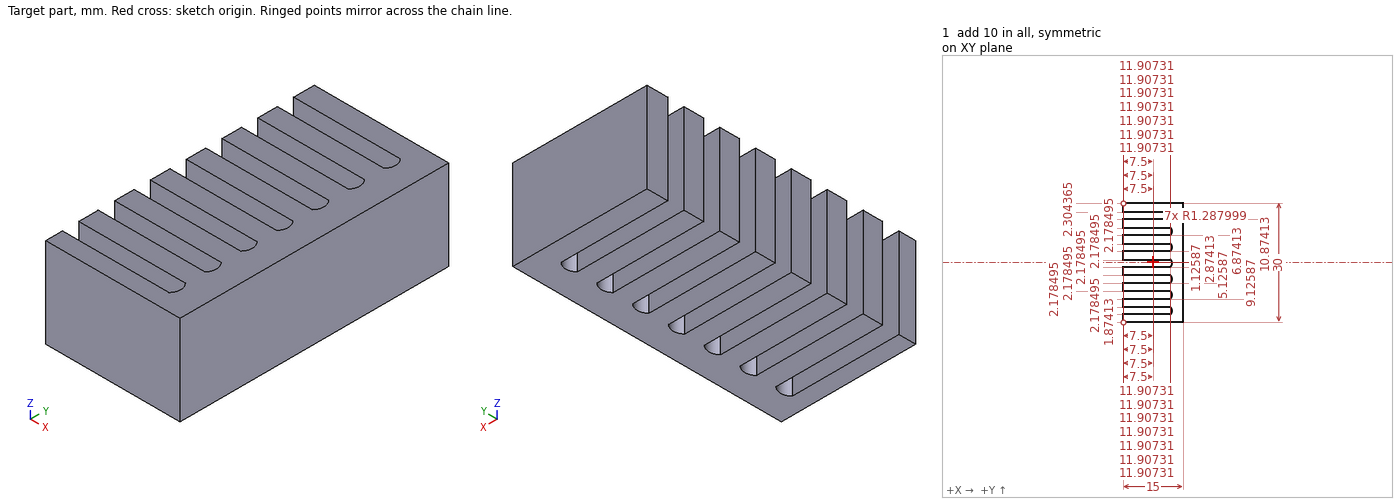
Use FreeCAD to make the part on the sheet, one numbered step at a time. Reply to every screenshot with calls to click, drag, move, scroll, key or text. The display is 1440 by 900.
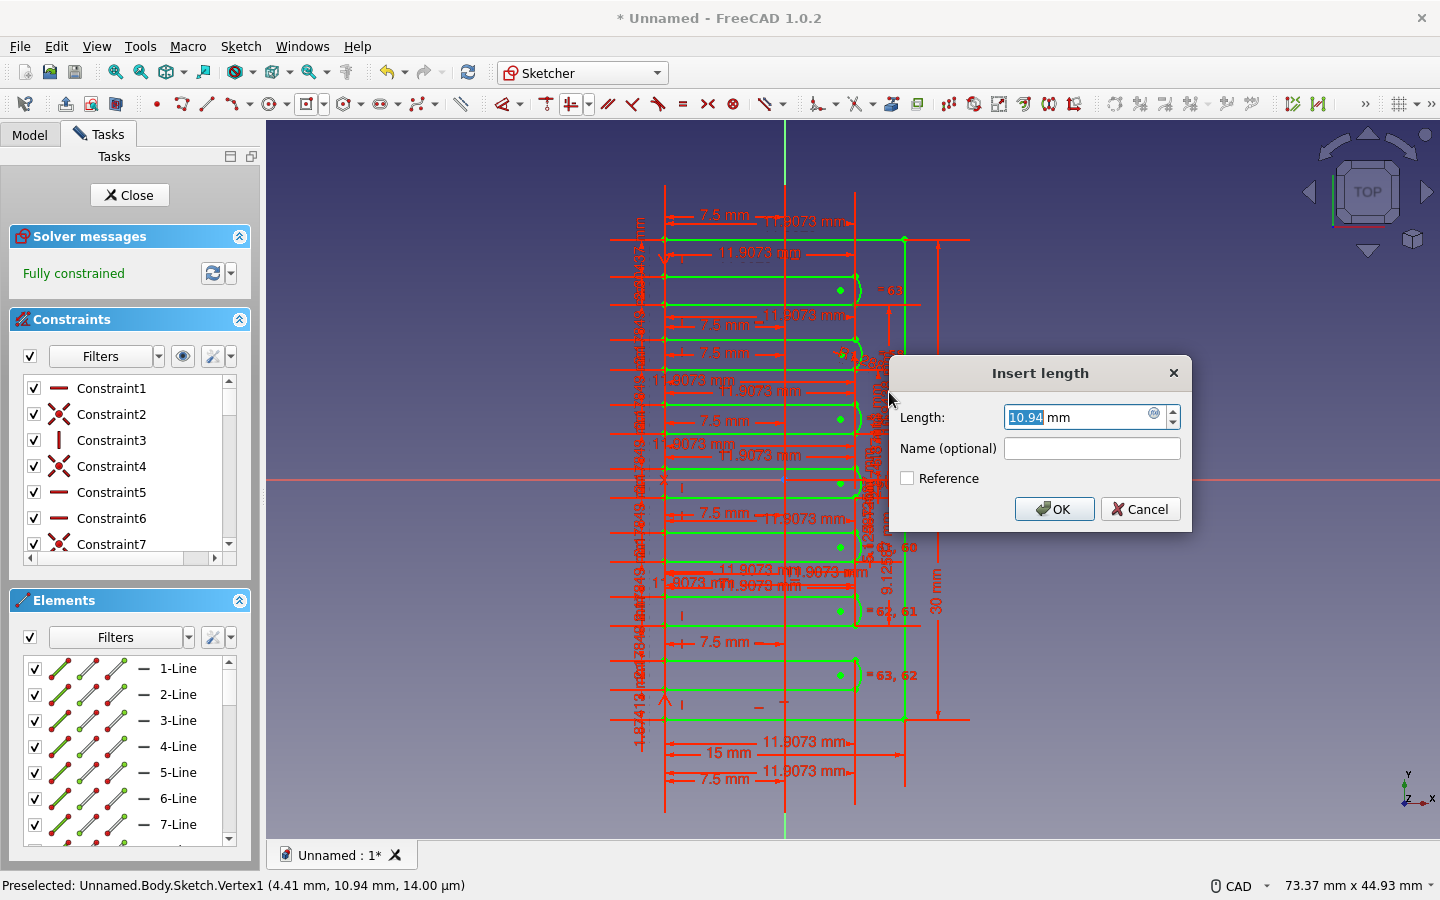
text(10.87413)
key(Return)
key(Escape)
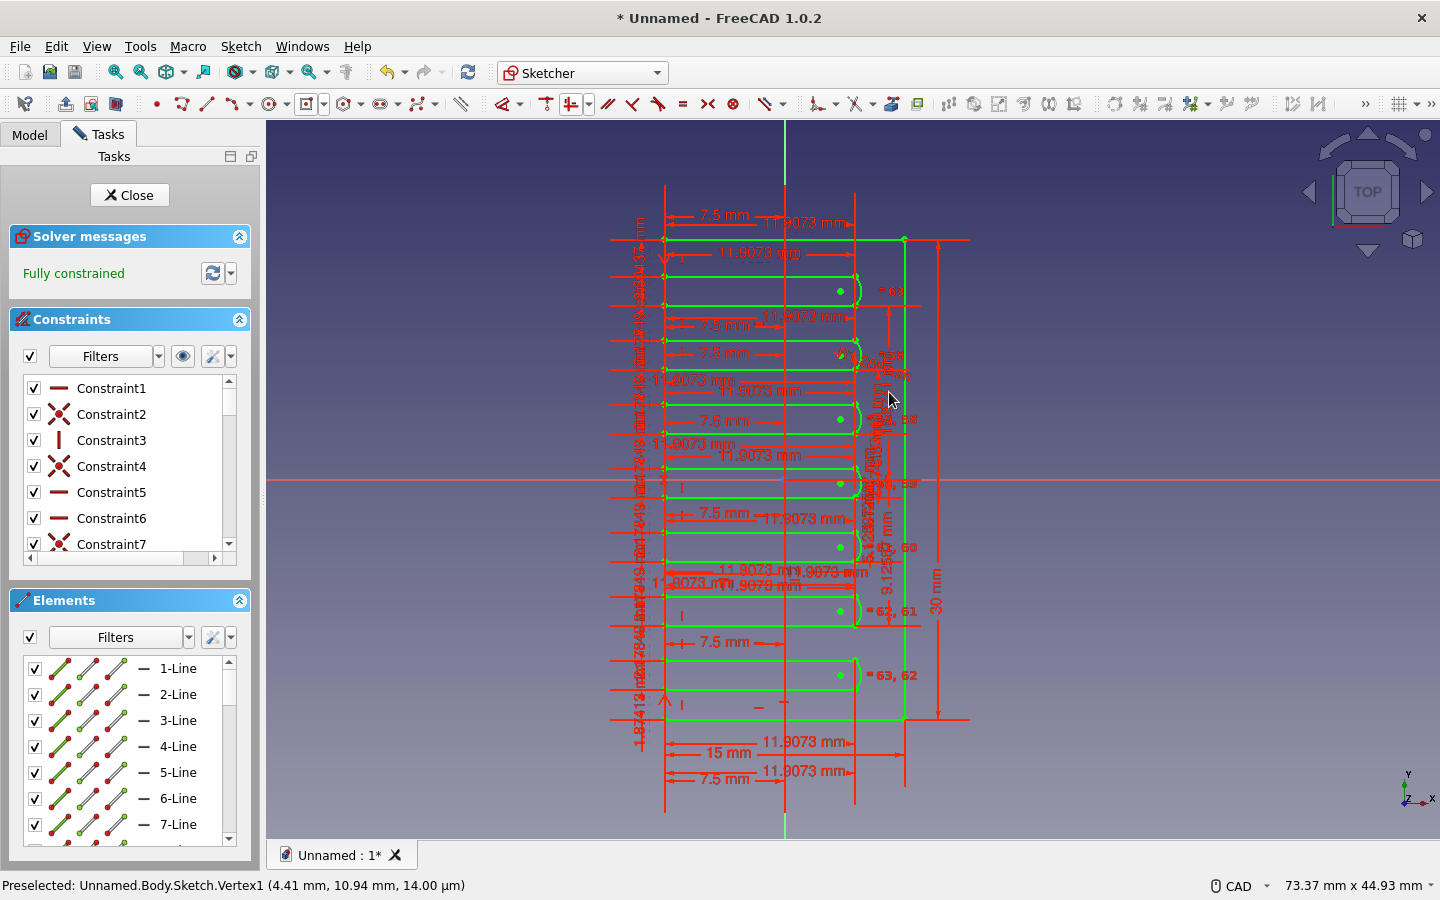
click(130, 195)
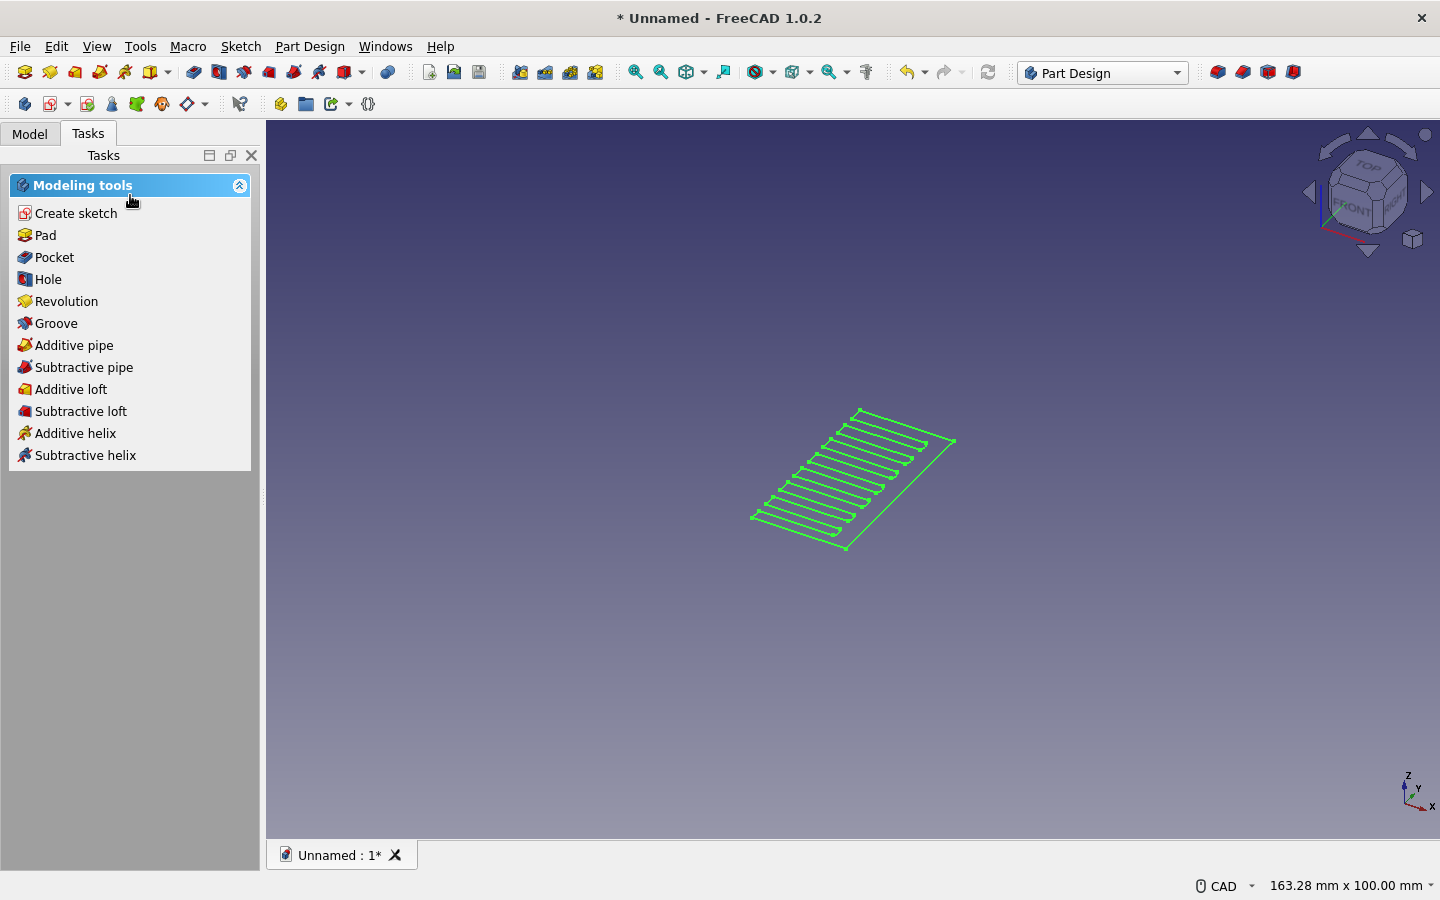
click(25, 72)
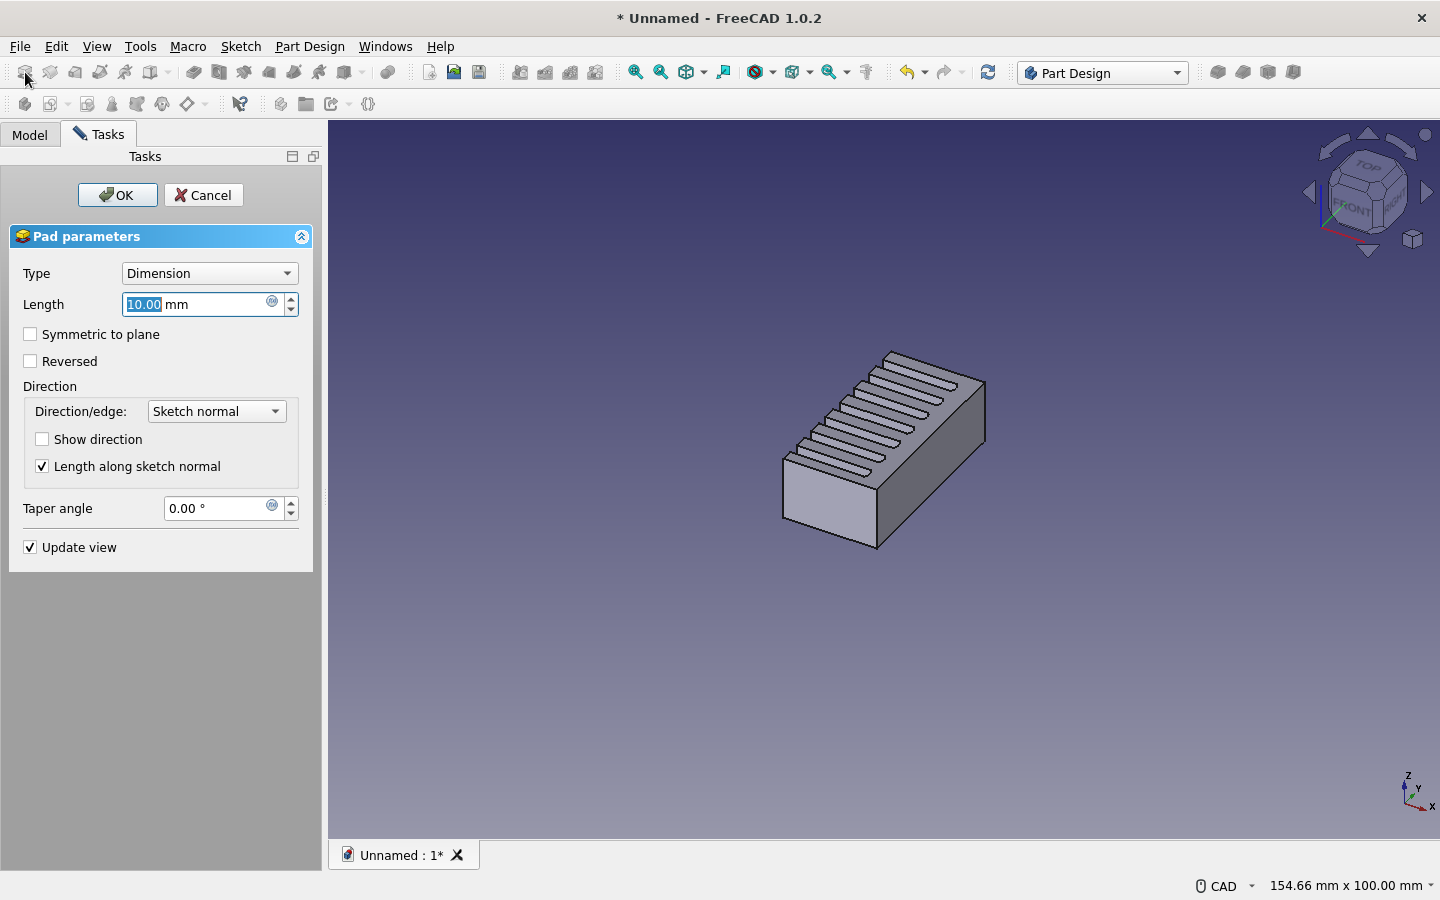
text(10)
key(Tab)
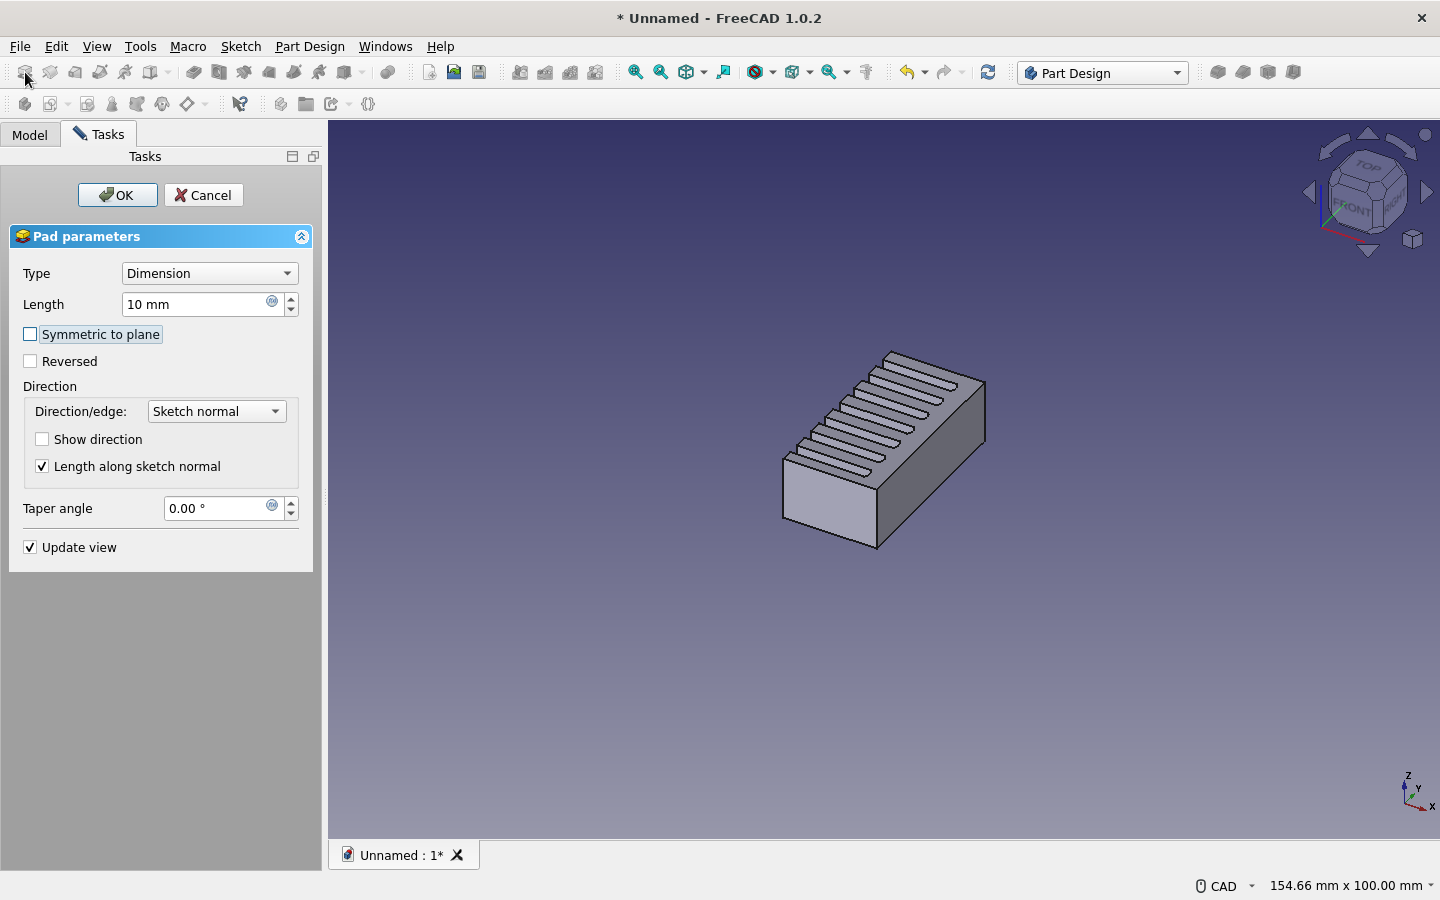
click(31, 334)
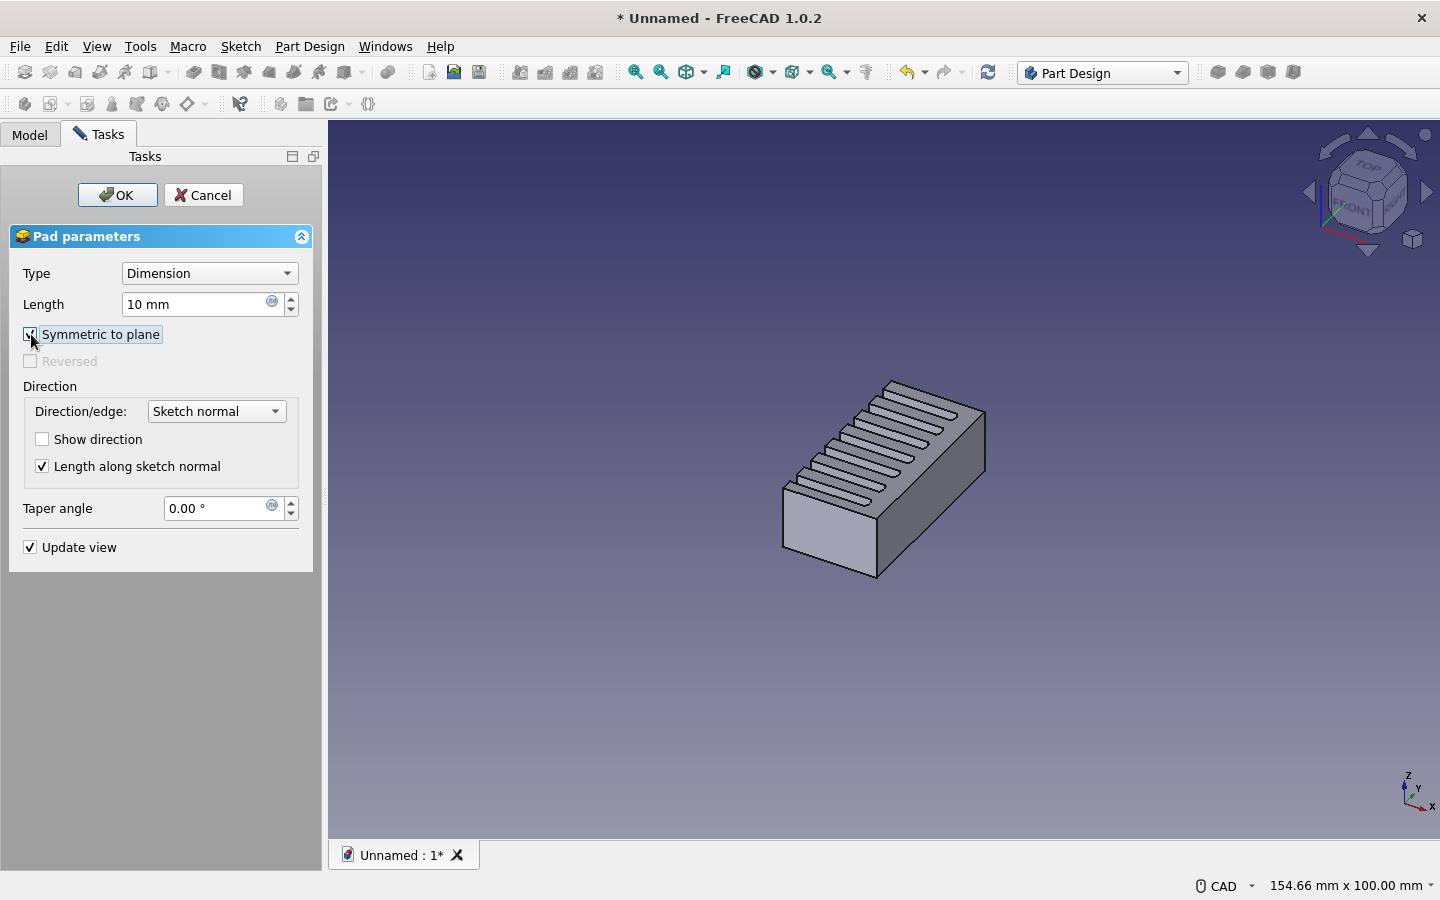
click(118, 195)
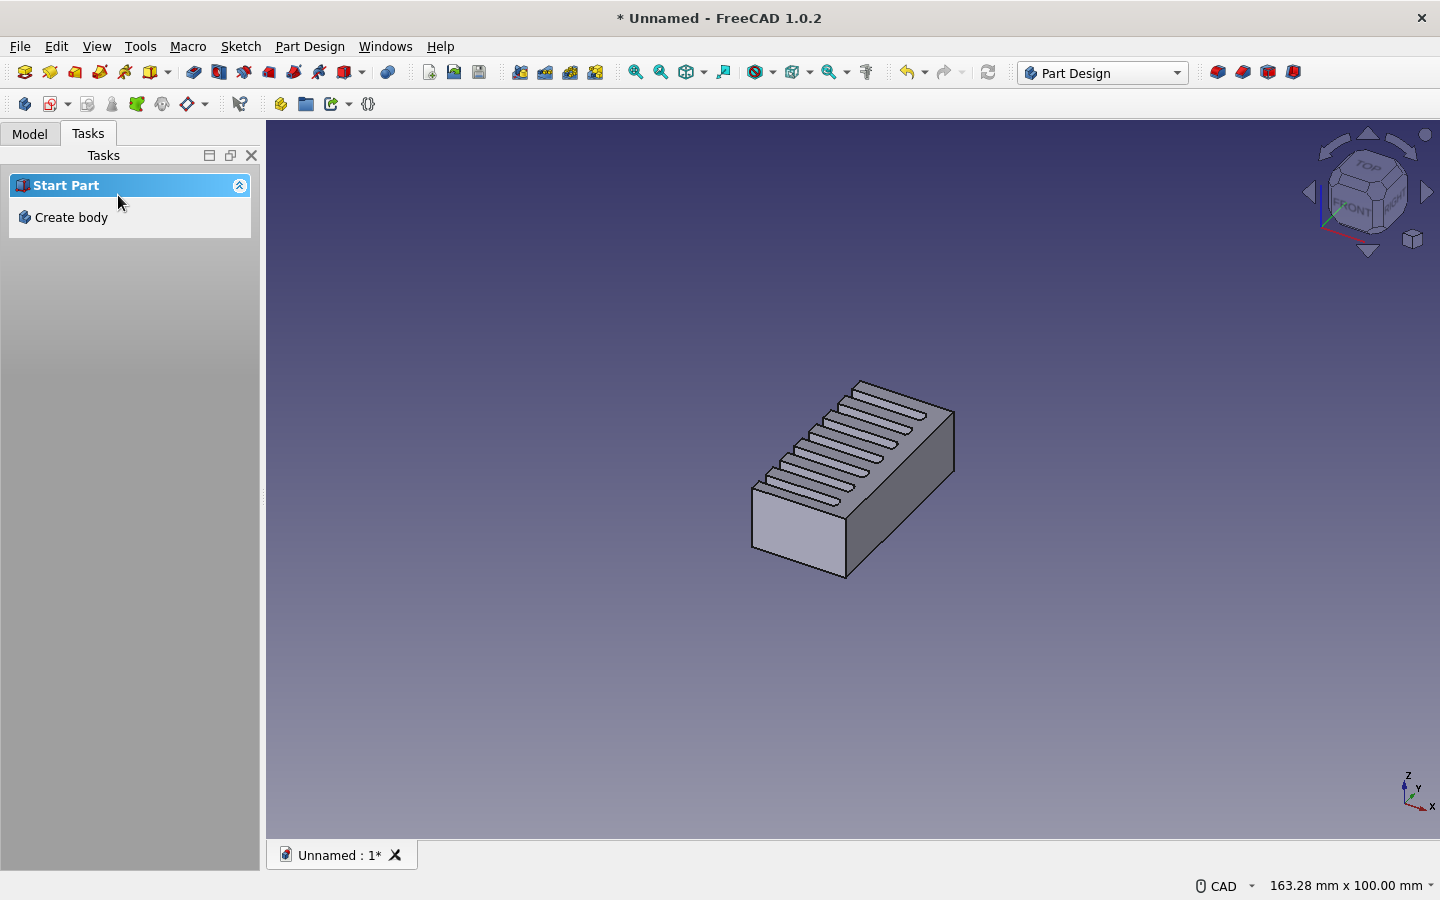
key(0)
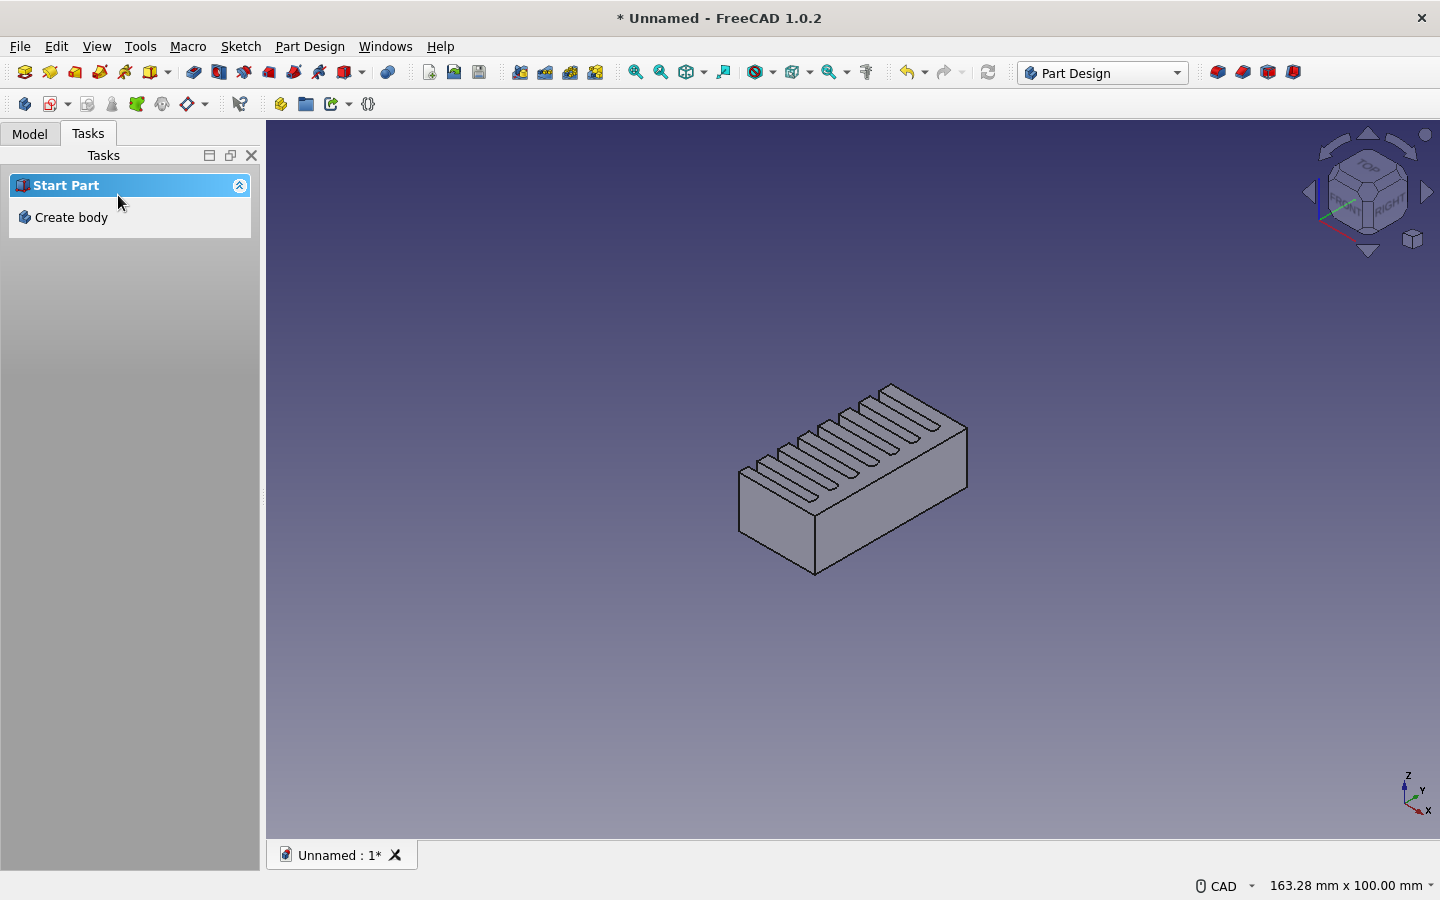
click(636, 72)